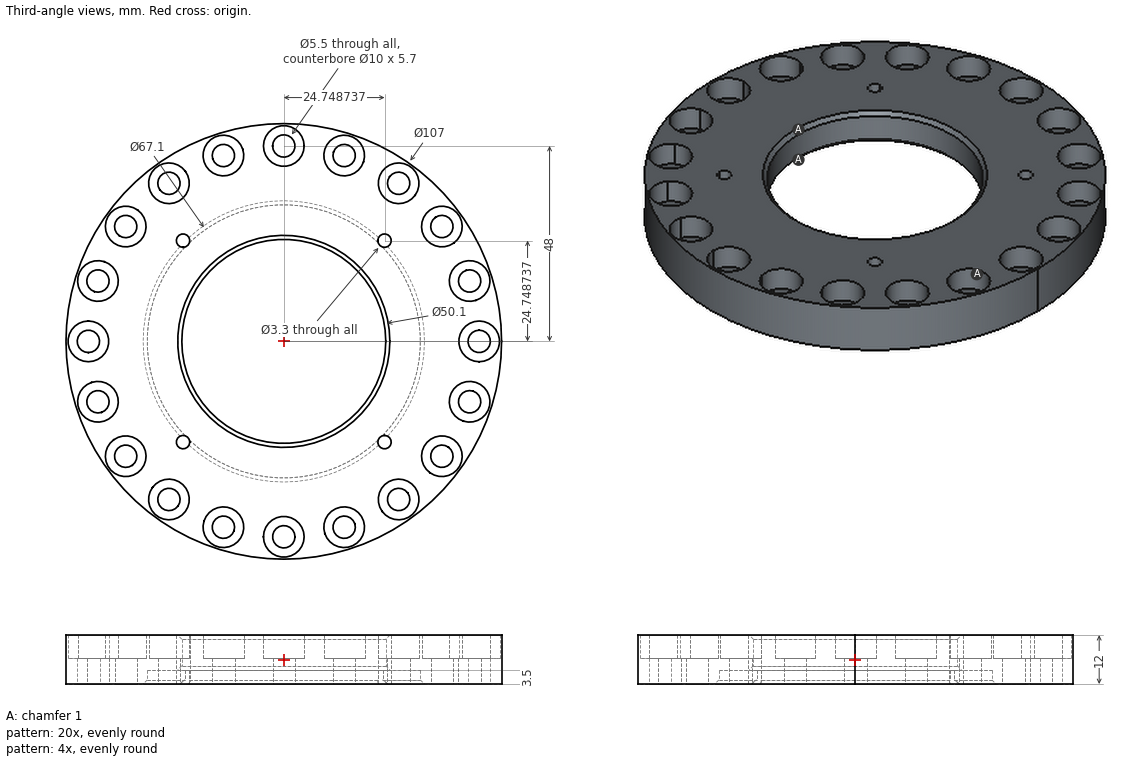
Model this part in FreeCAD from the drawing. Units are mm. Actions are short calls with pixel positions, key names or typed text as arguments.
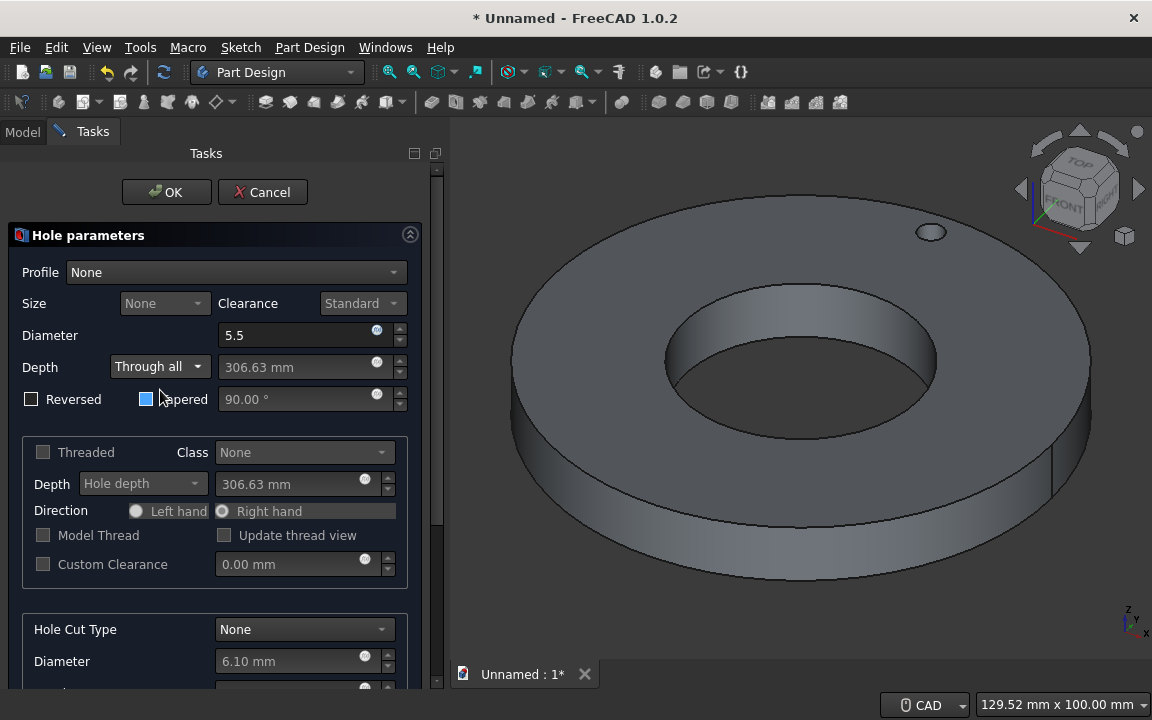
click(306, 630)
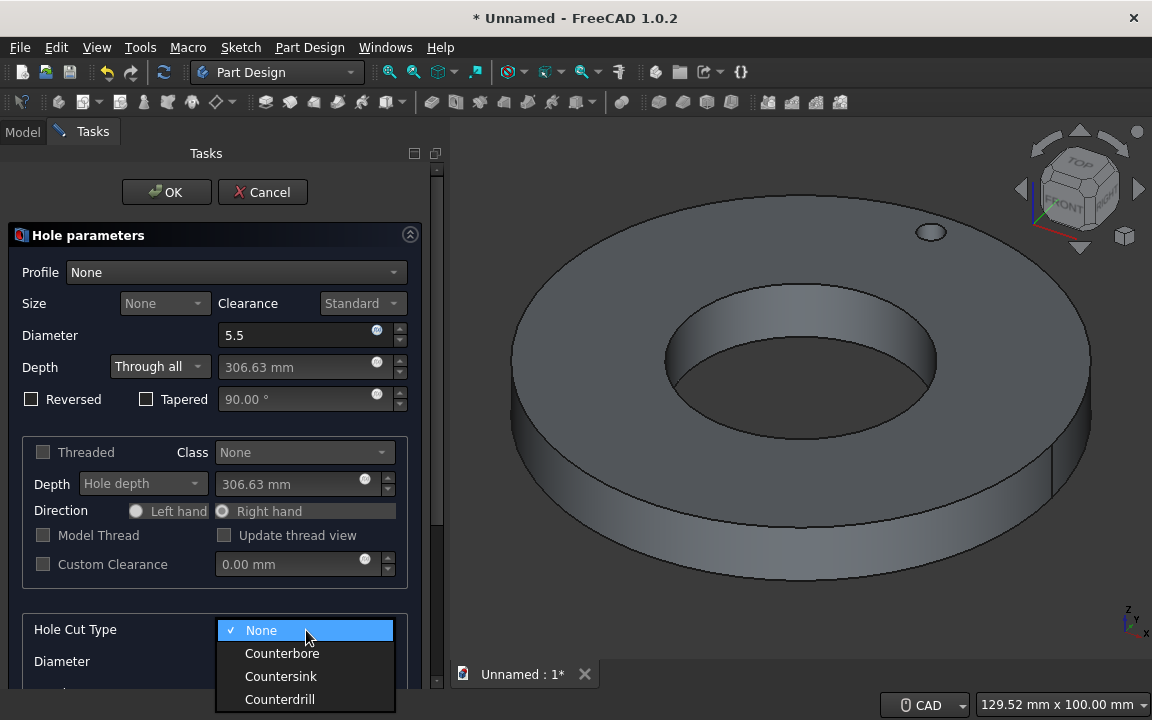
click(304, 654)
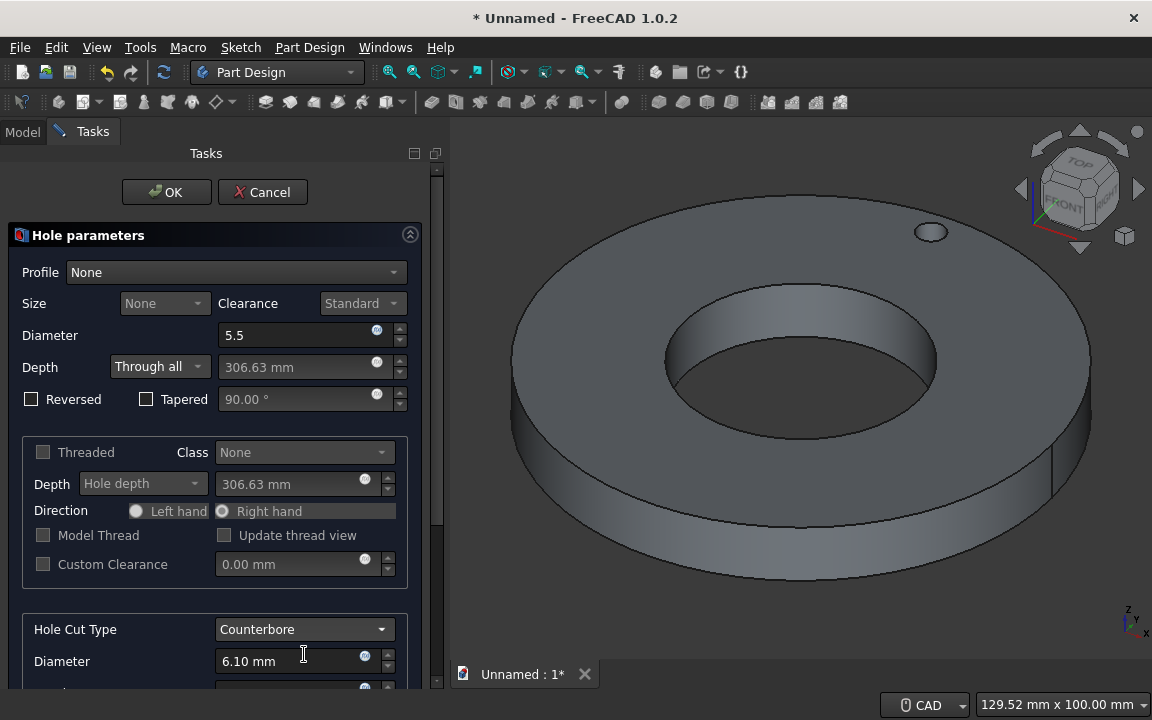
triple_click(298, 661)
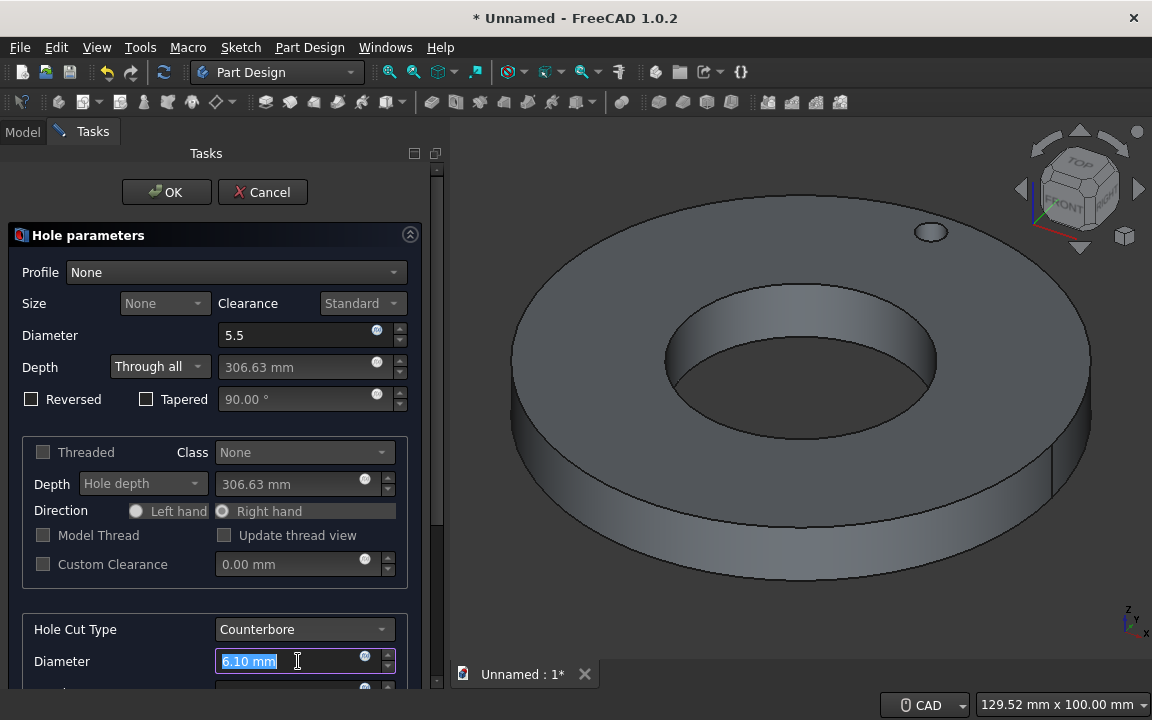
text(10)
key(Tab)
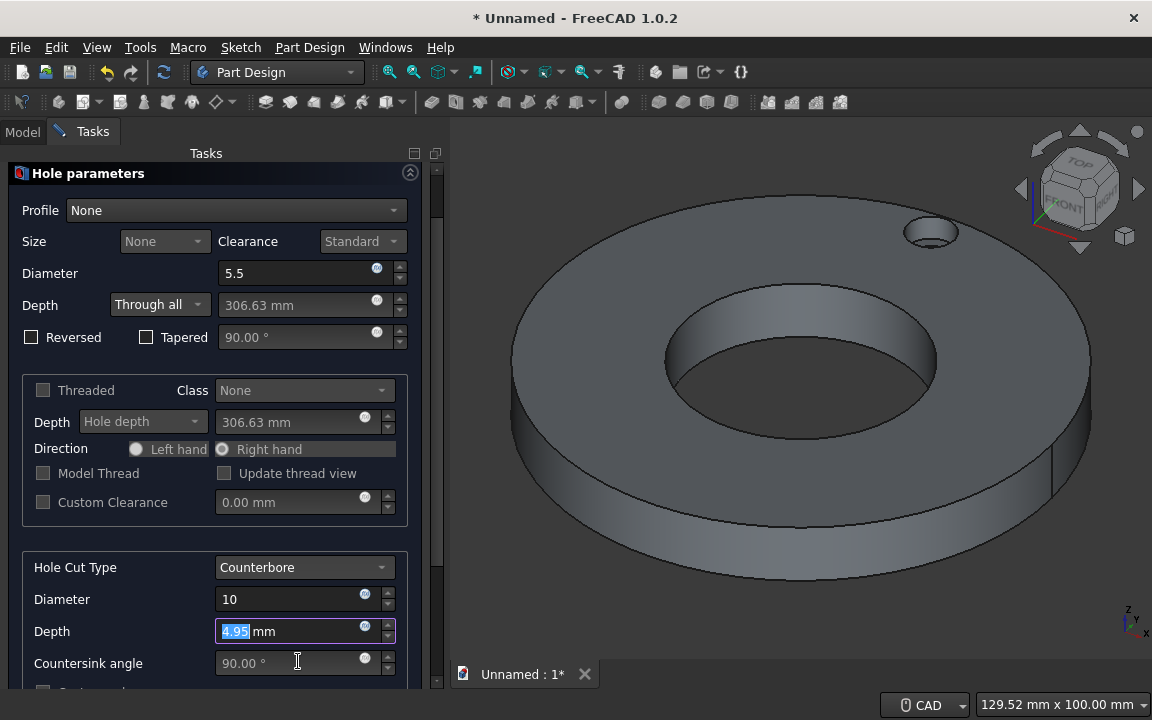
text(5.7)
key(Tab)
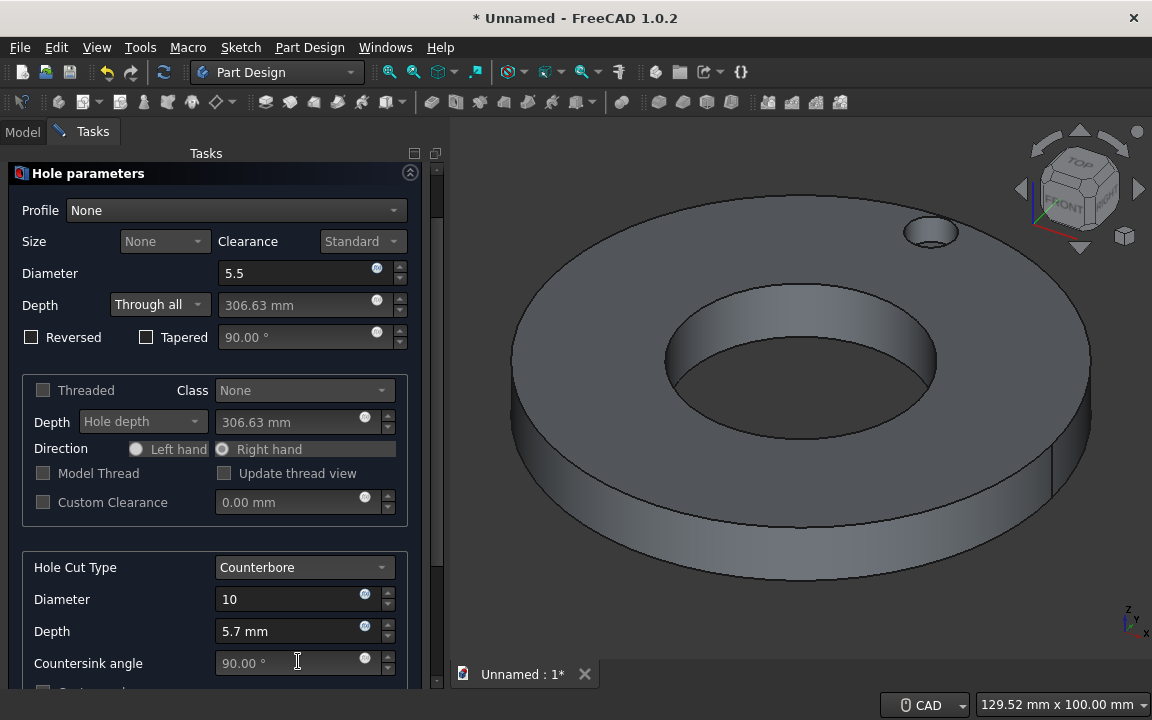
scroll(437, 426, up, 2)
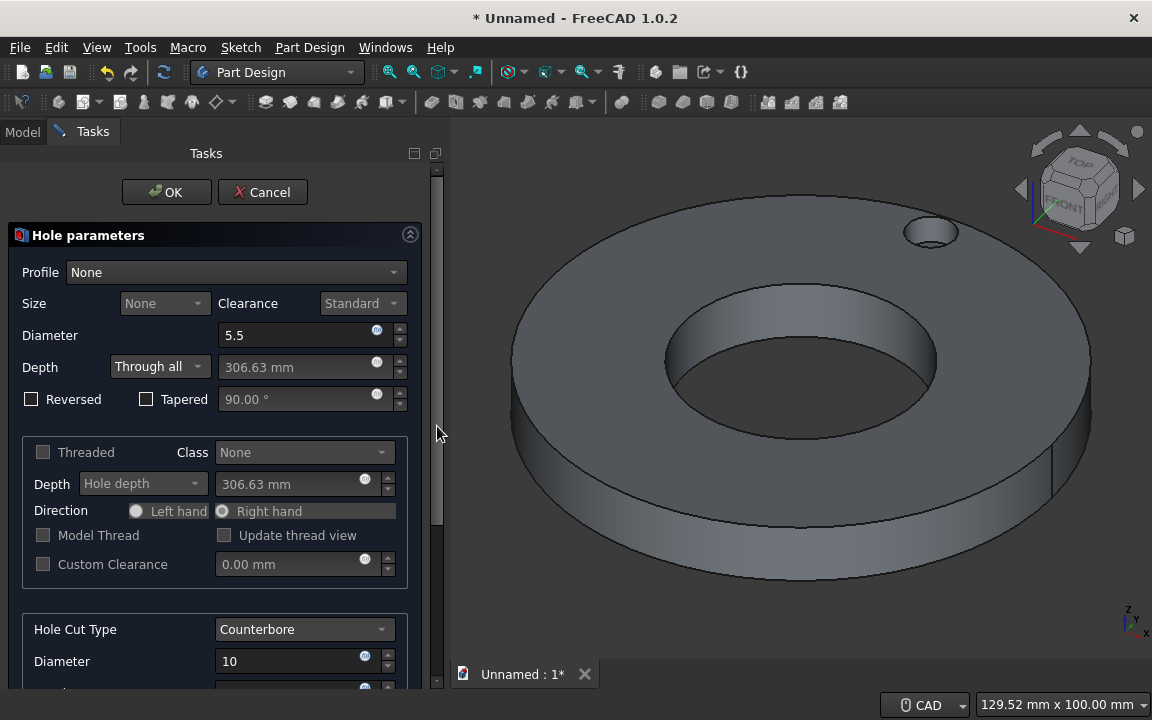
click(167, 192)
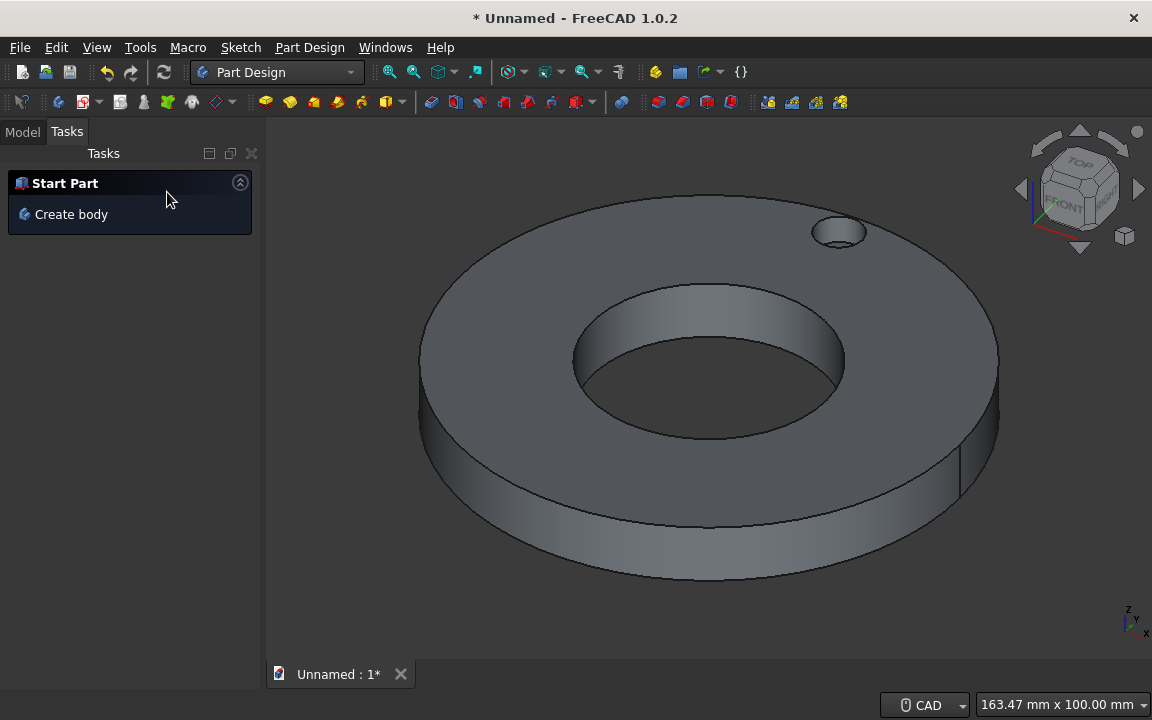
key(5)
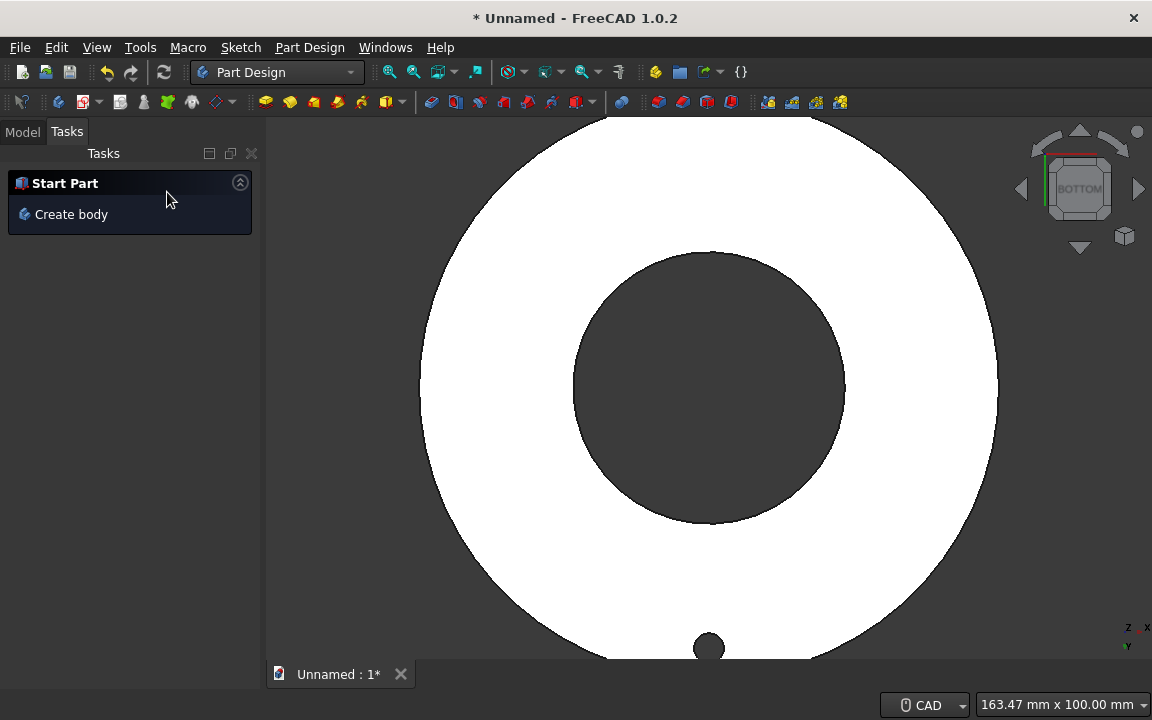
key(v)
key(f)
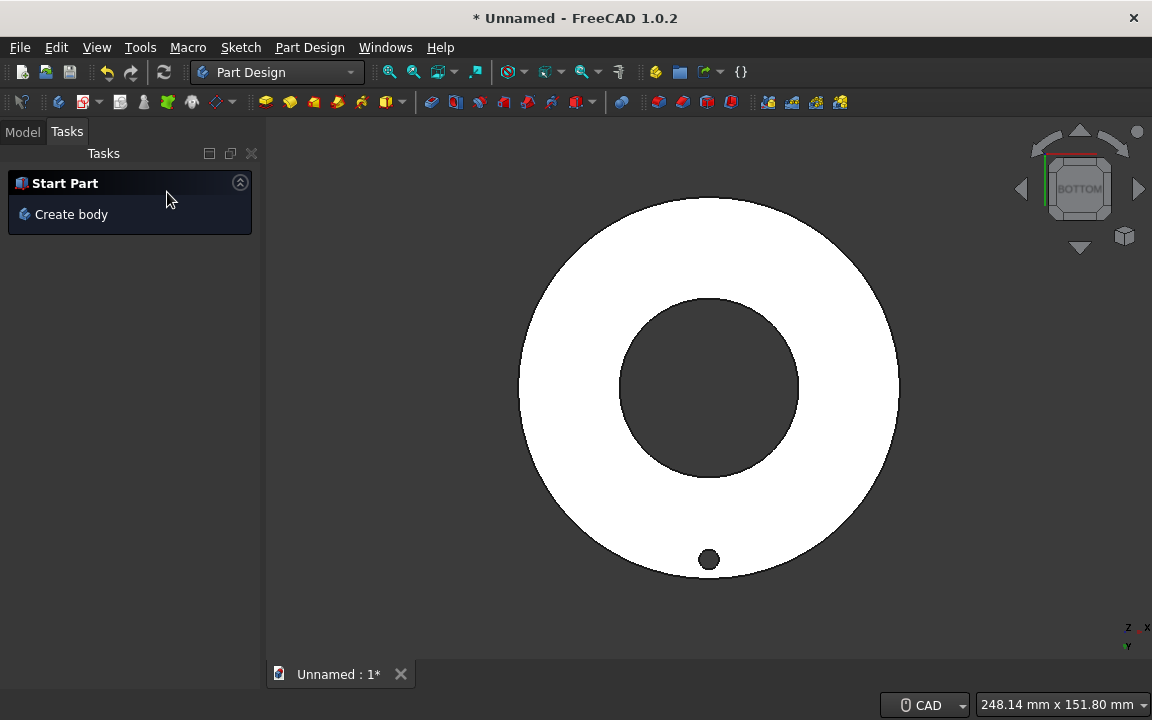
click(818, 496)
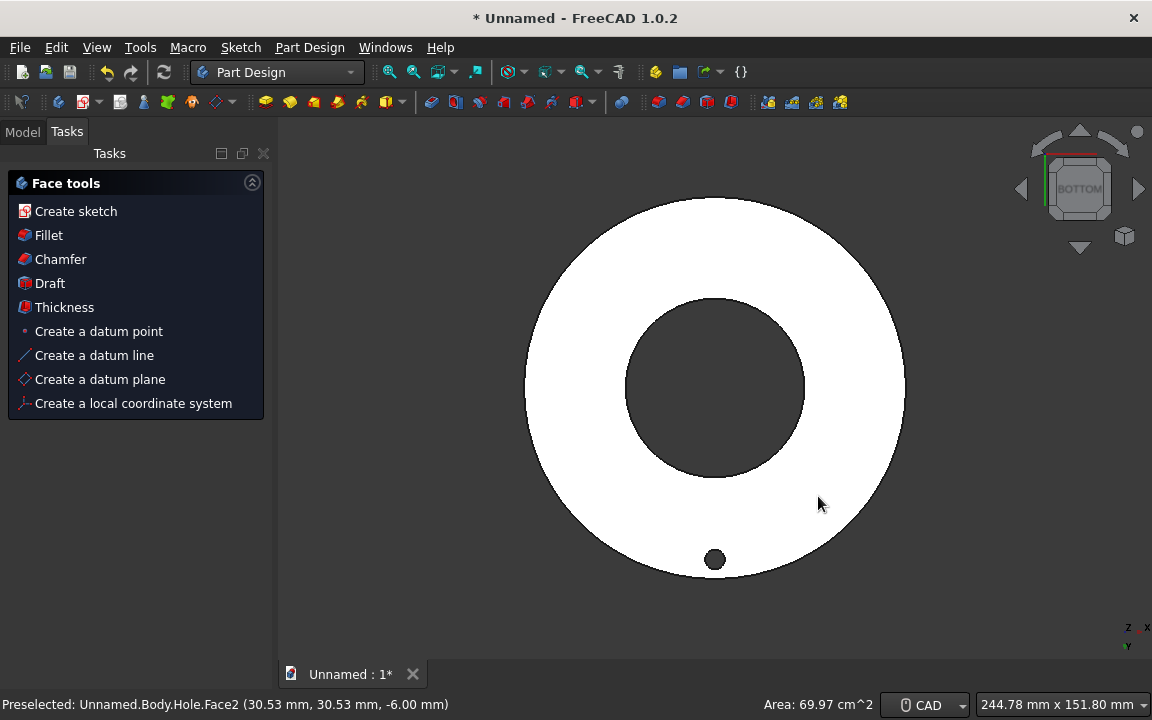
click(84, 102)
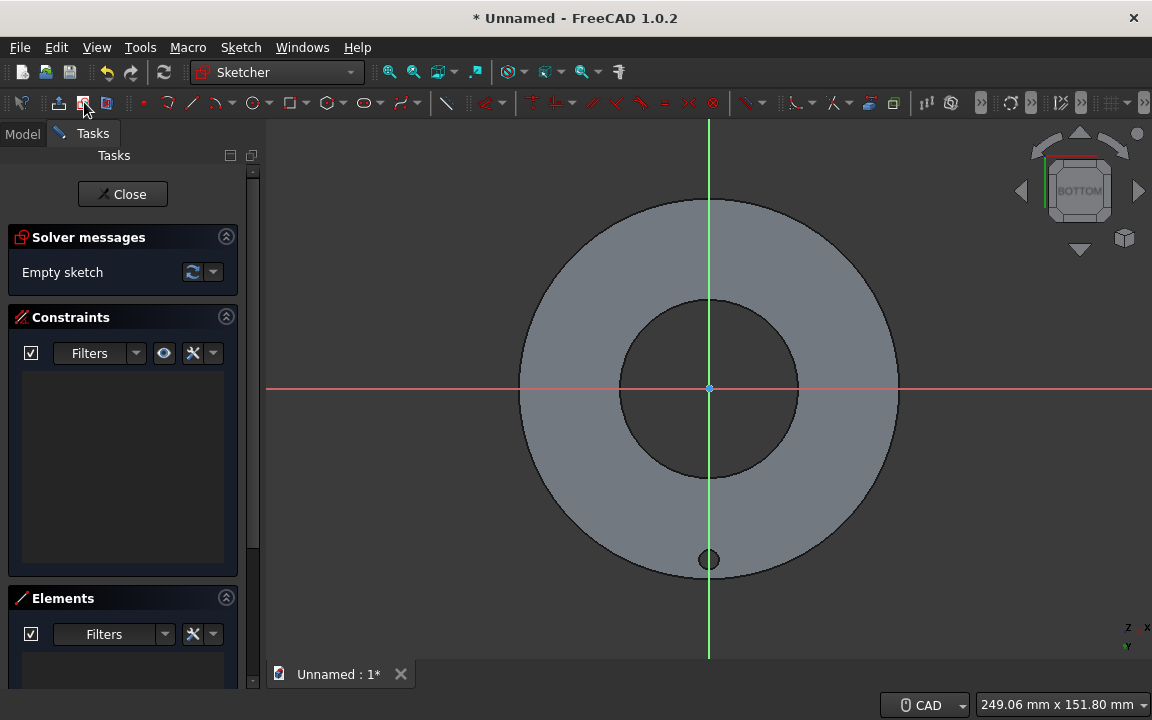
scroll(848, 389, up, 2)